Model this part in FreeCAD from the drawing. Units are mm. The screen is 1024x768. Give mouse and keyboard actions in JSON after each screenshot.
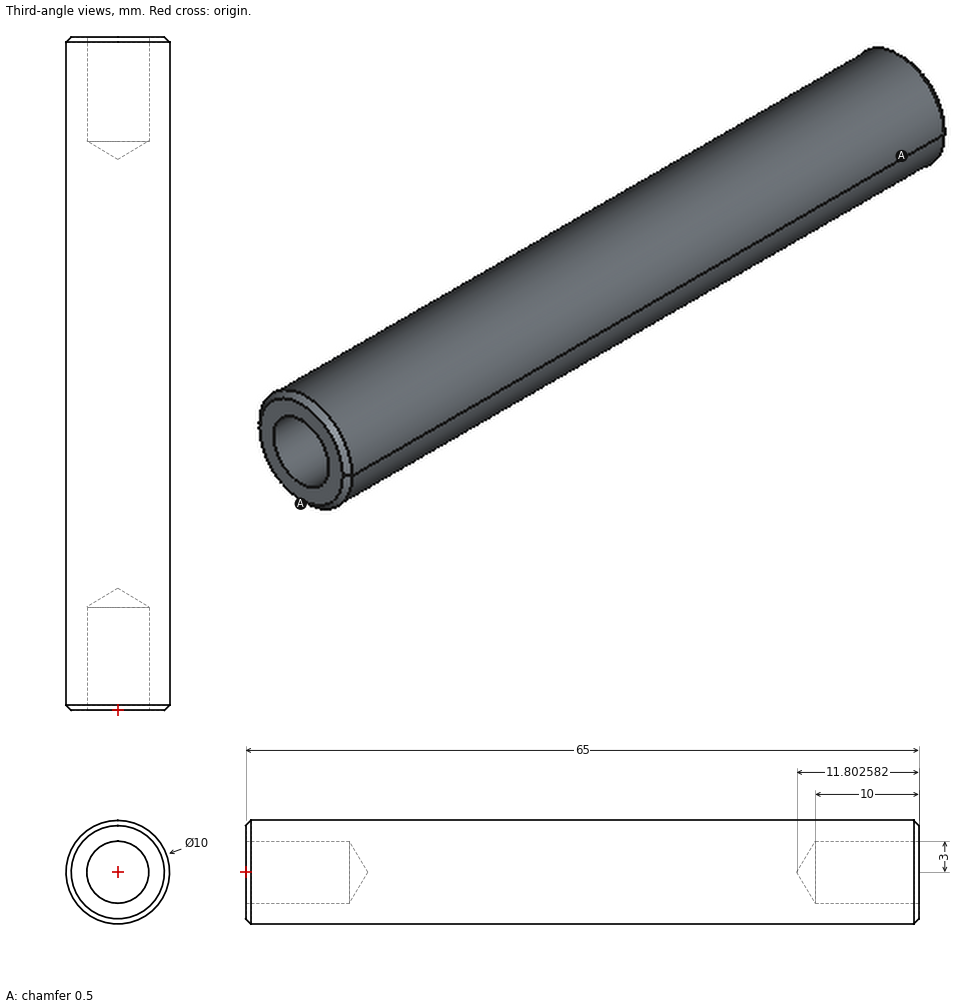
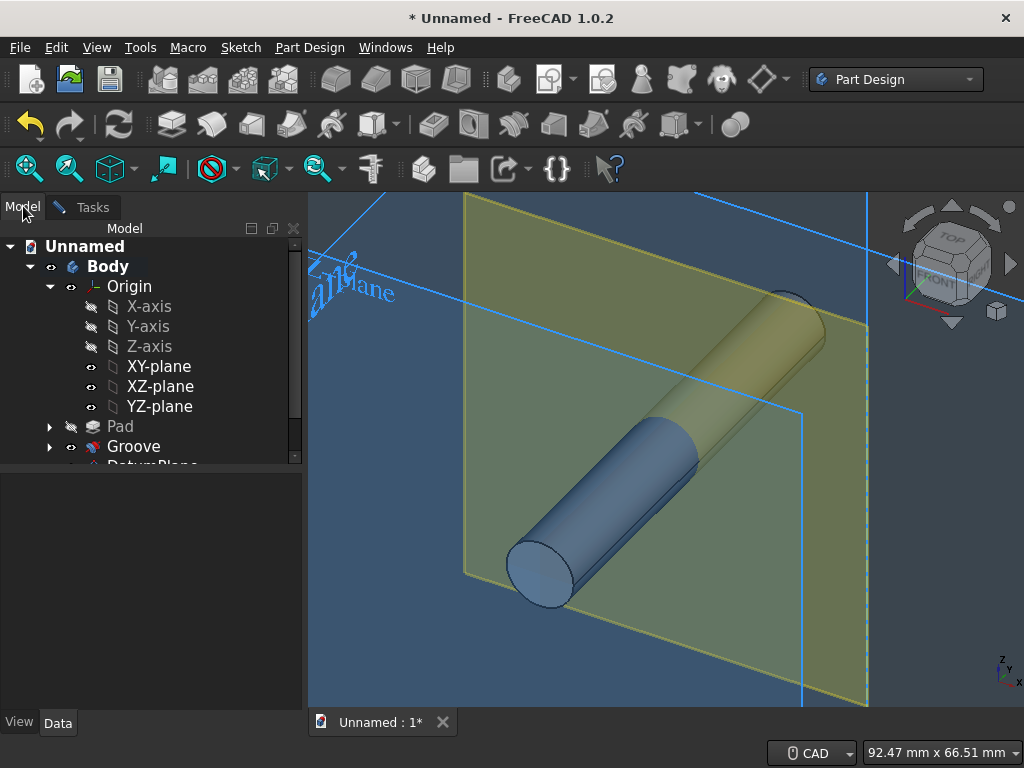
{"action": "scroll", "coordinate": [100, 342], "scroll_direction": "down", "scroll_amount": 3}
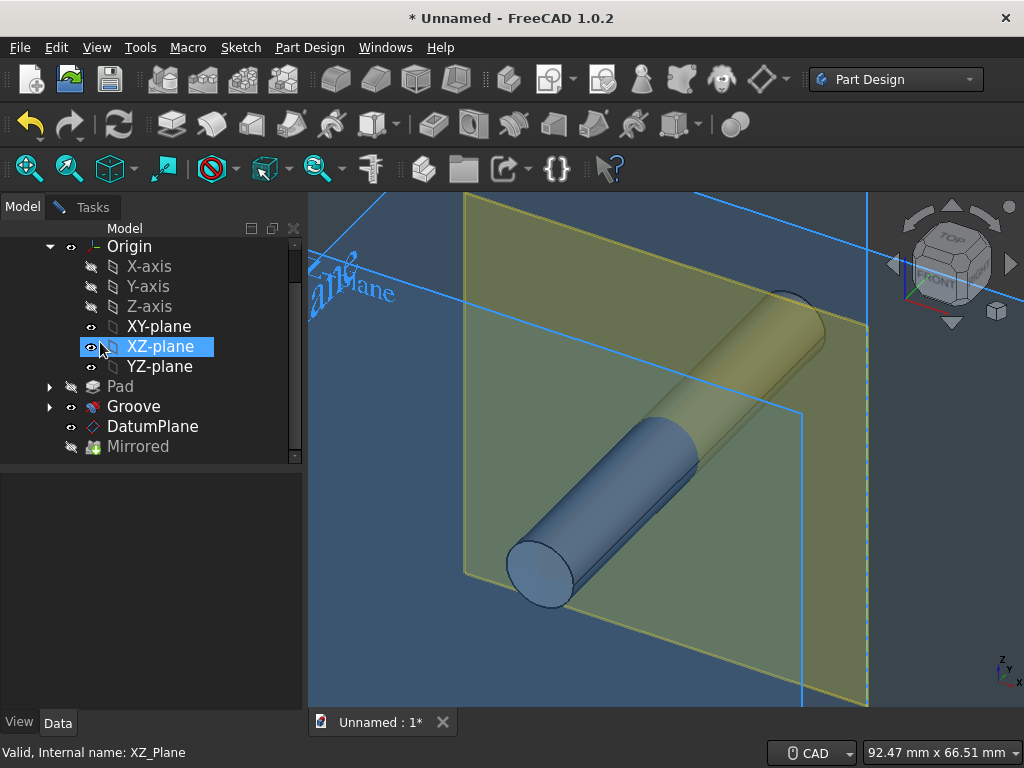
{"action": "left_click", "coordinate": [116, 427]}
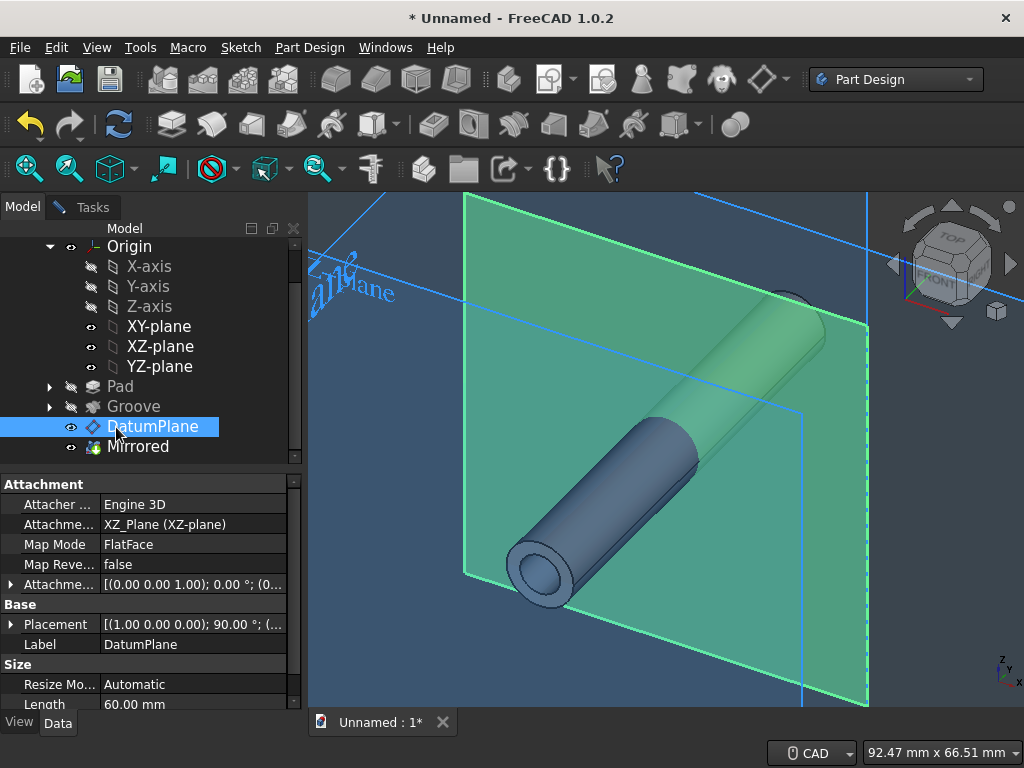
{"action": "left_click", "coordinate": [84, 206]}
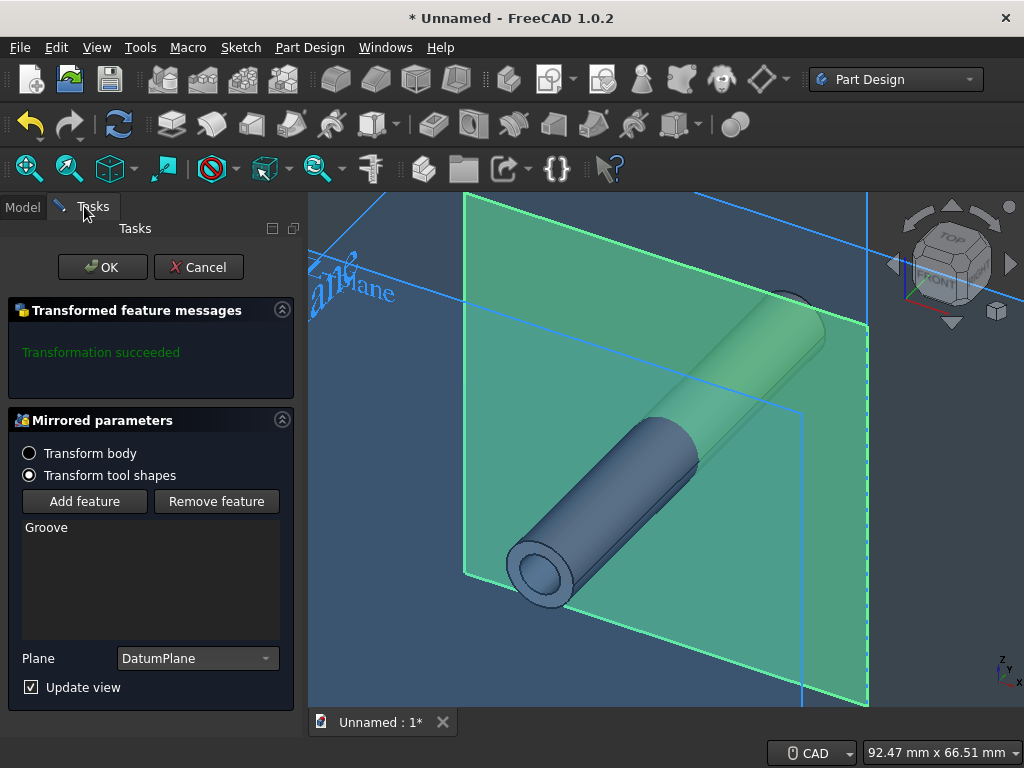
{"action": "left_click", "coordinate": [103, 267]}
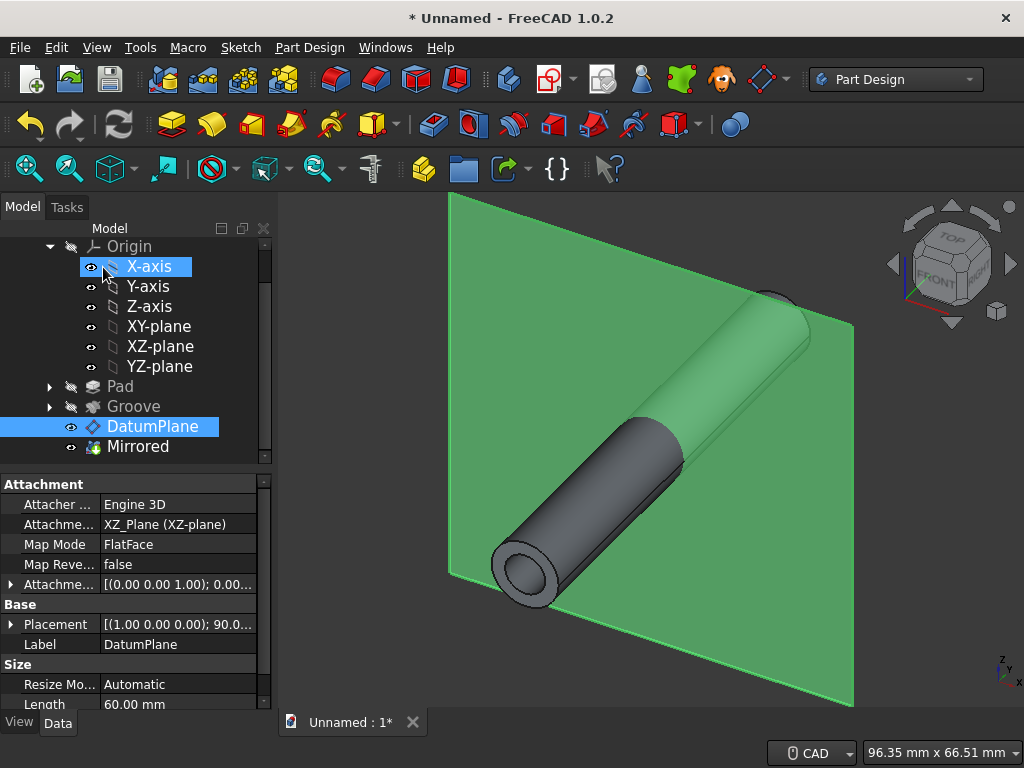
{"action": "left_click", "coordinate": [116, 427]}
{"action": "key", "text": "space"}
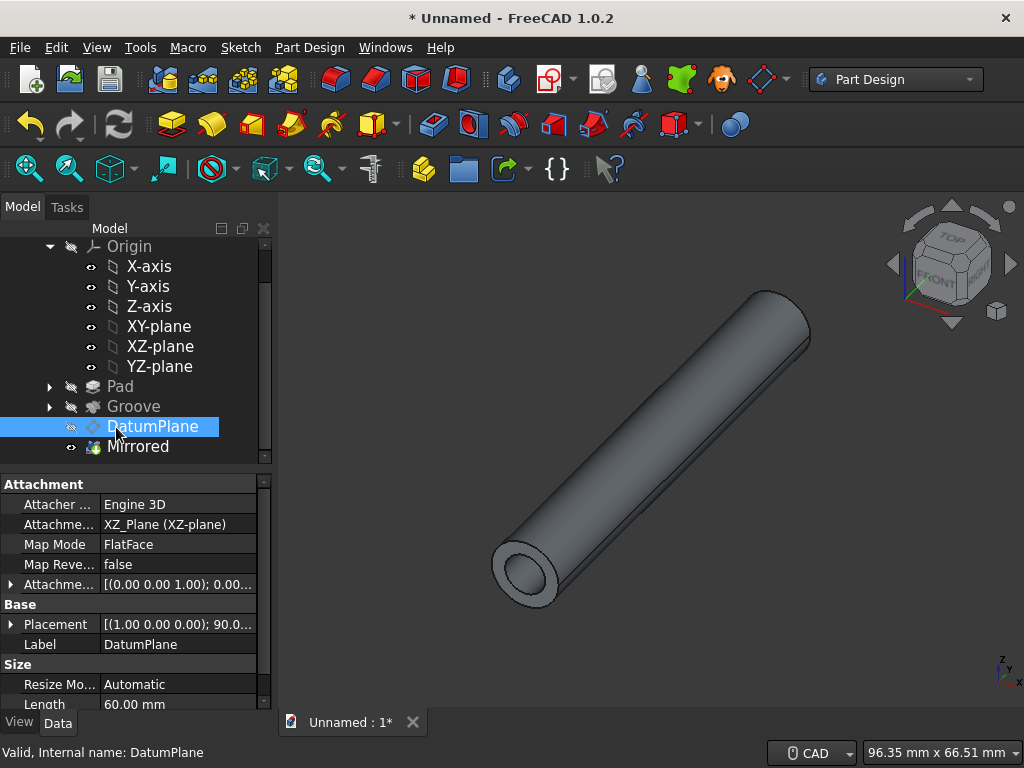
{"action": "left_click", "coordinate": [498, 546]}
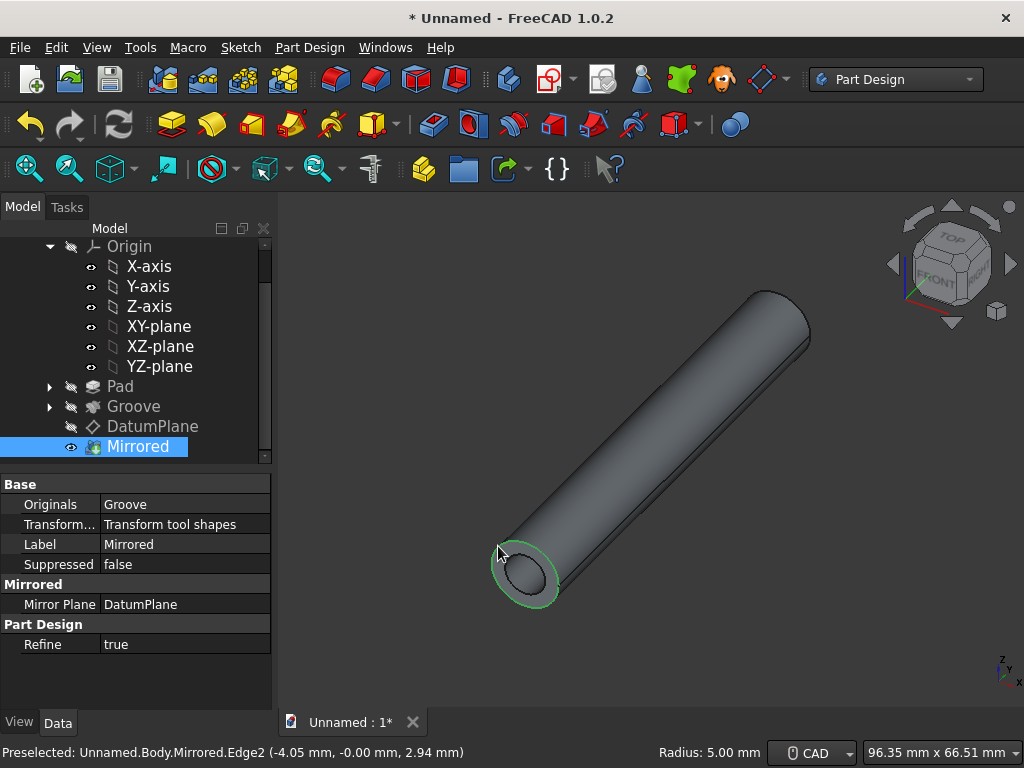
{"action": "key", "text": "0"}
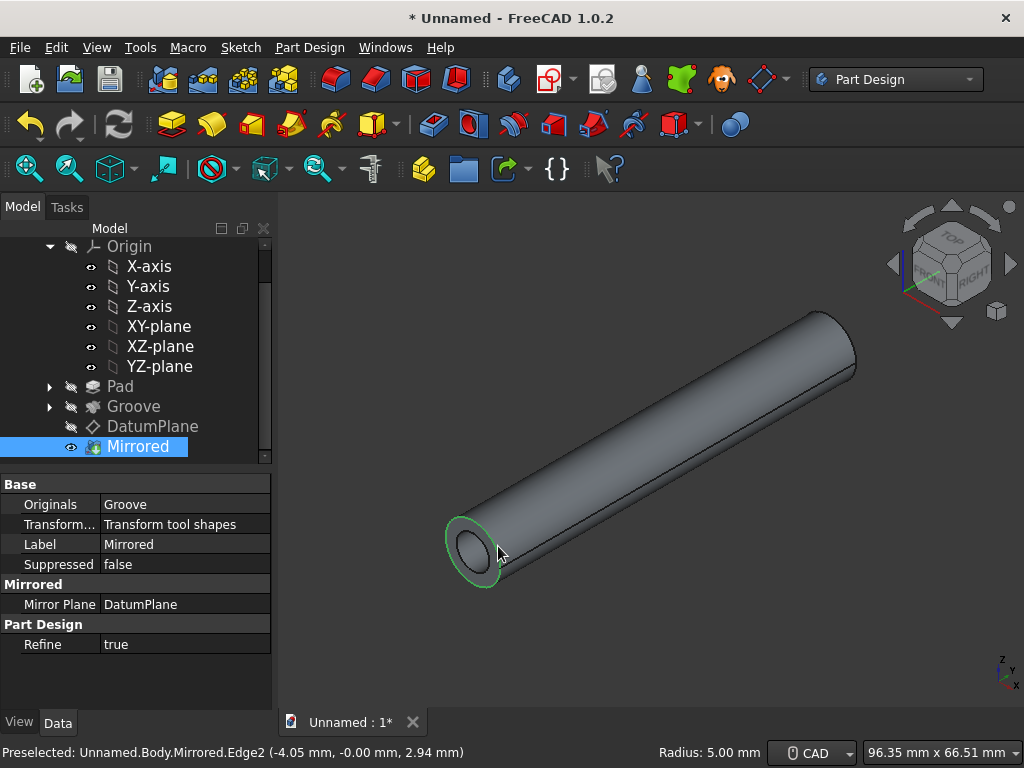
{"action": "key", "text": "2"}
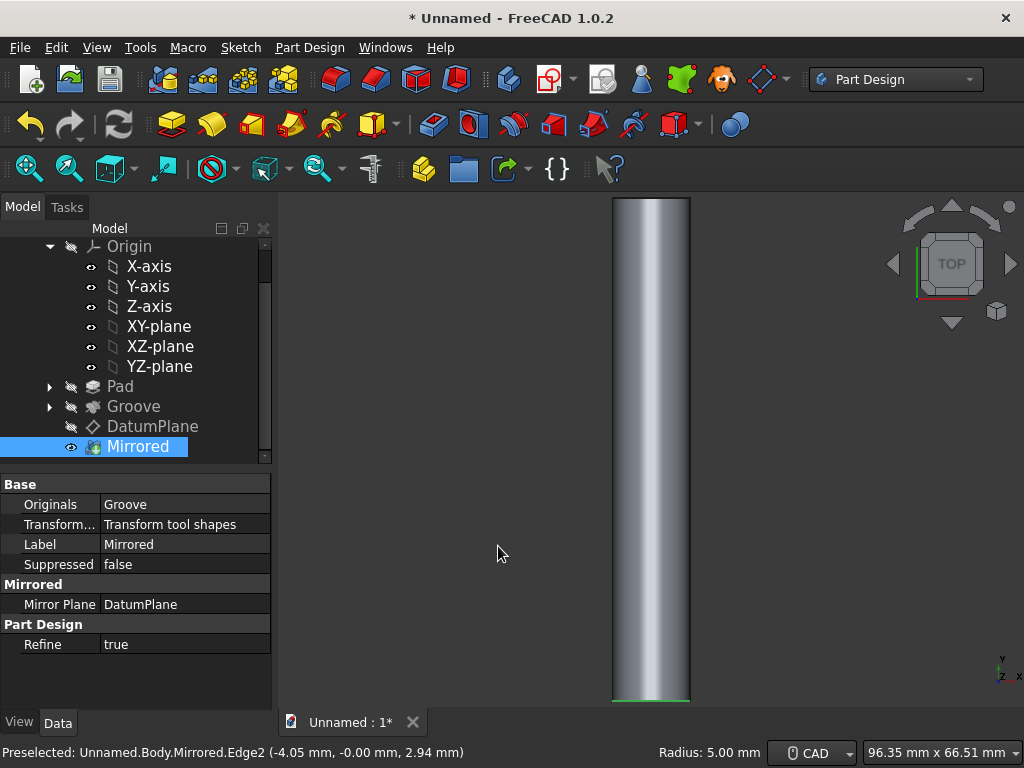
{"action": "key", "text": "1"}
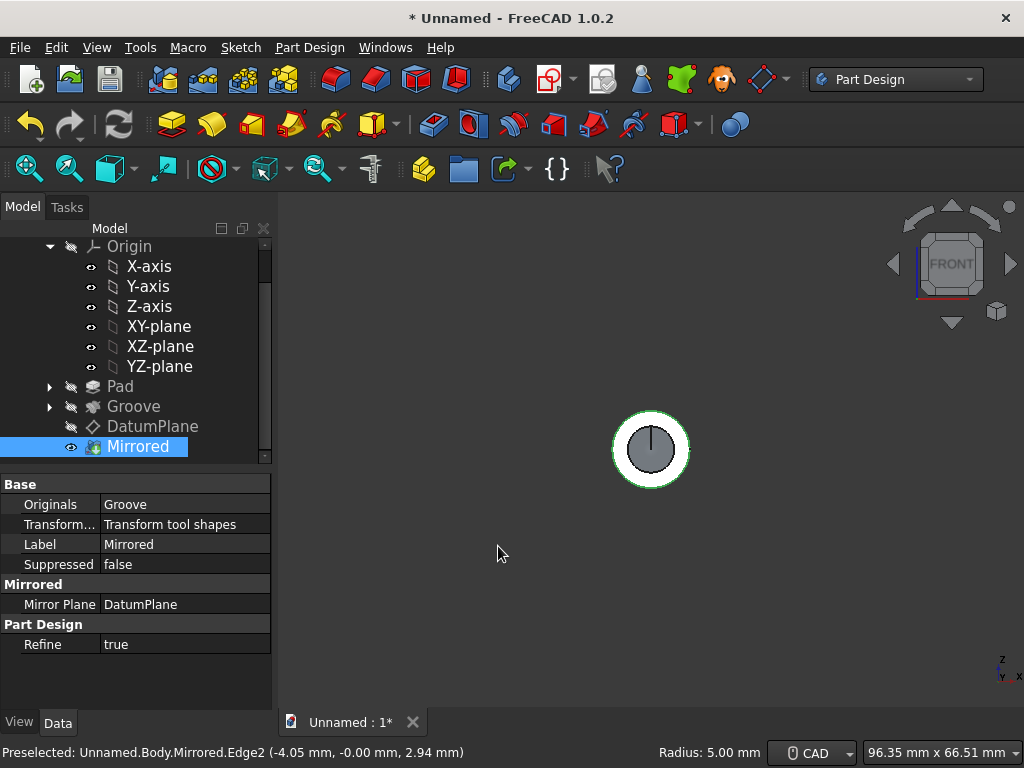
{"action": "left_click", "coordinate": [30, 170]}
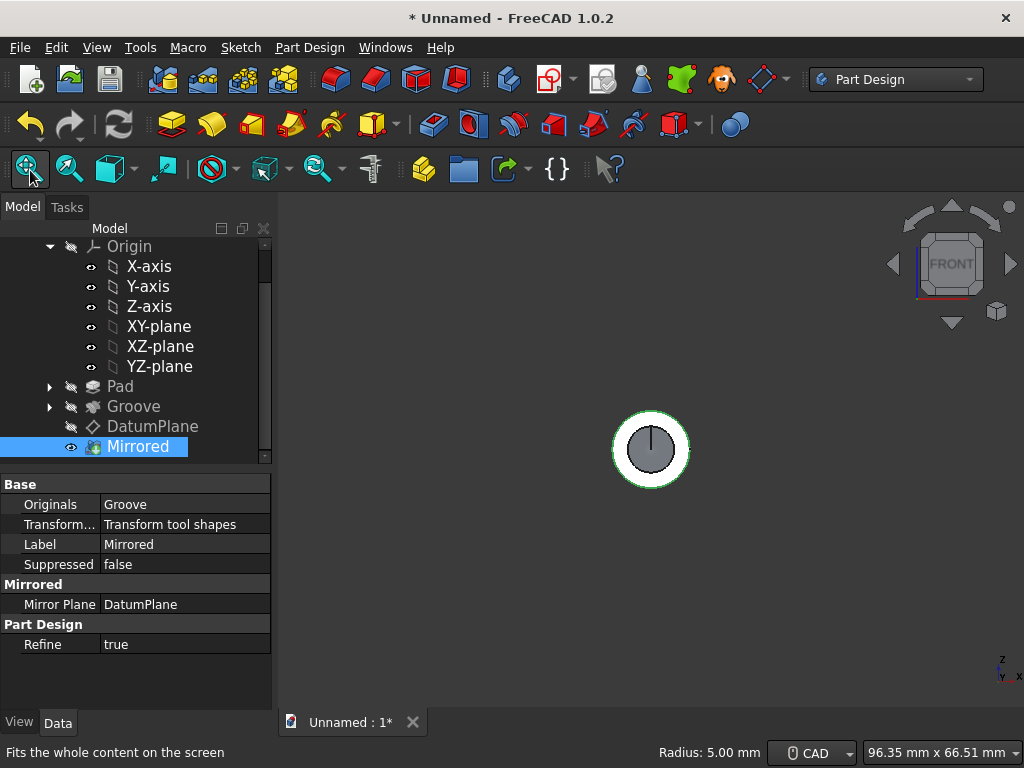
{"action": "key", "text": "3"}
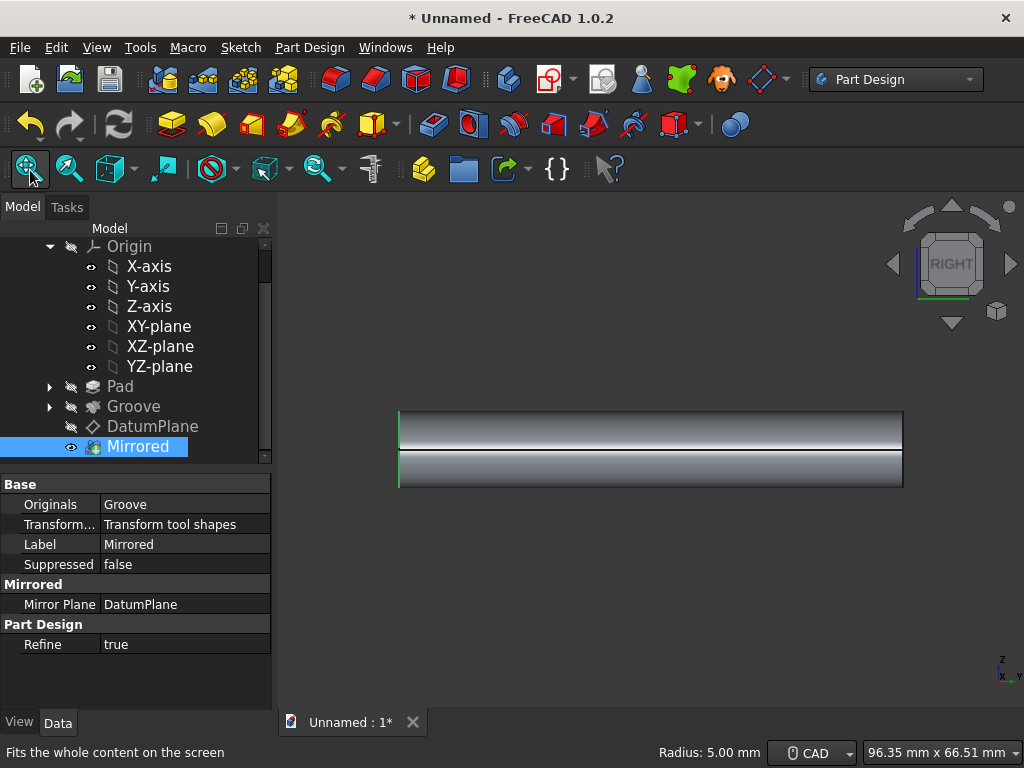
{"action": "left_click", "coordinate": [903, 426], "text": "ctrl"}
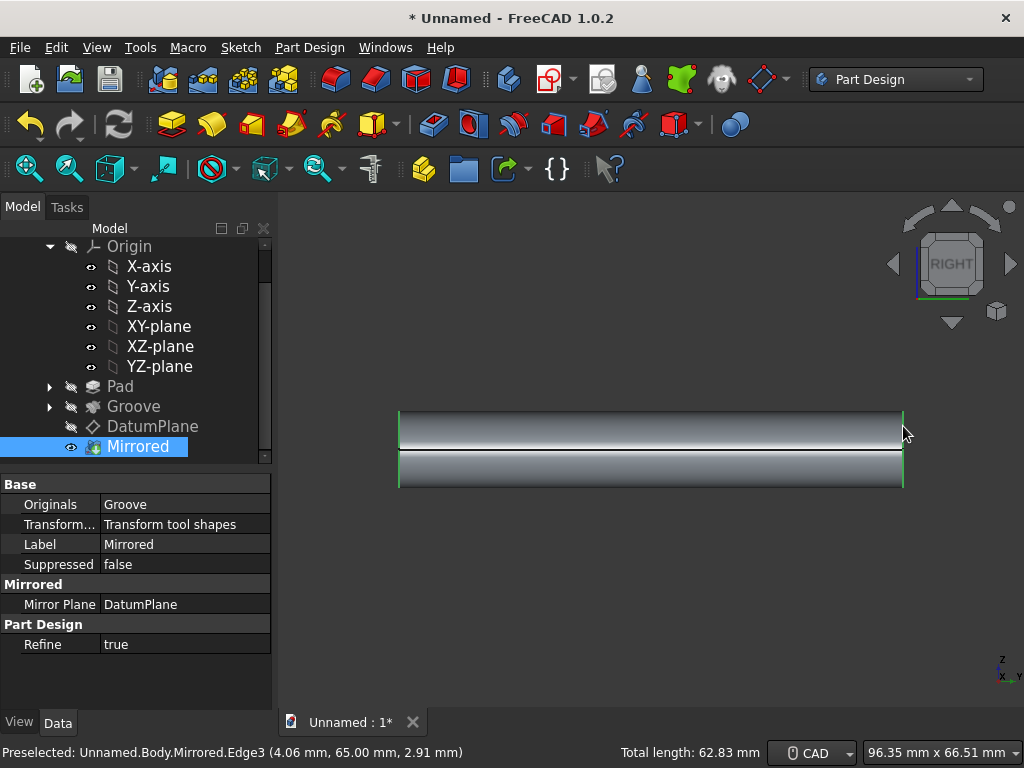
{"action": "left_click", "coordinate": [376, 80]}